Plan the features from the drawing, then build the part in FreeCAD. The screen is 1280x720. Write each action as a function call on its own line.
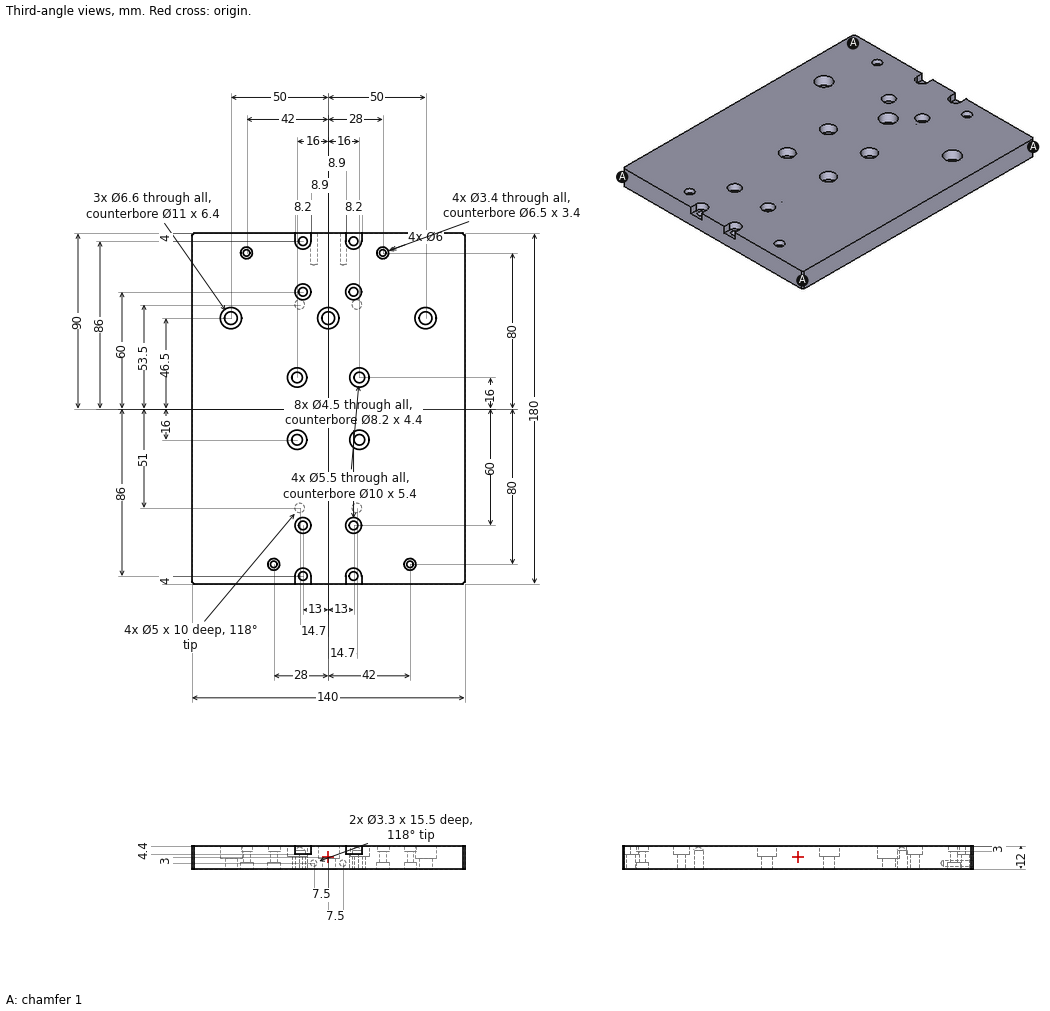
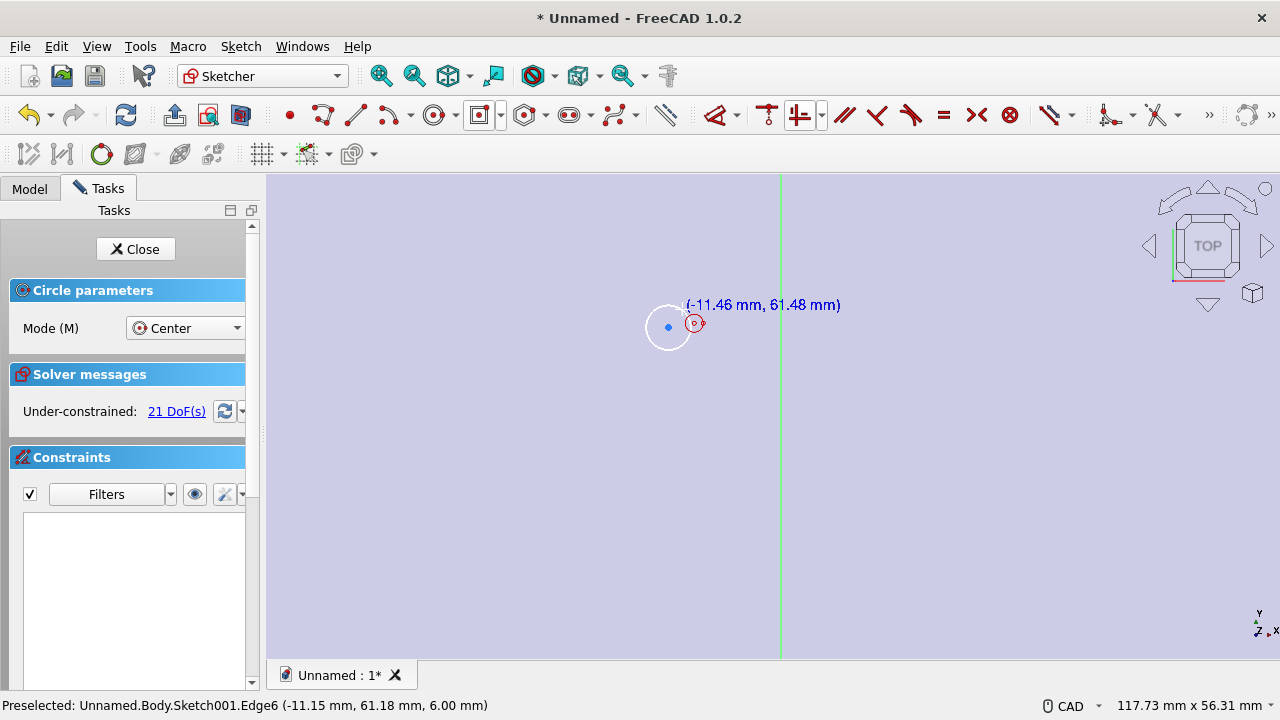
scroll(685, 309, down, 8)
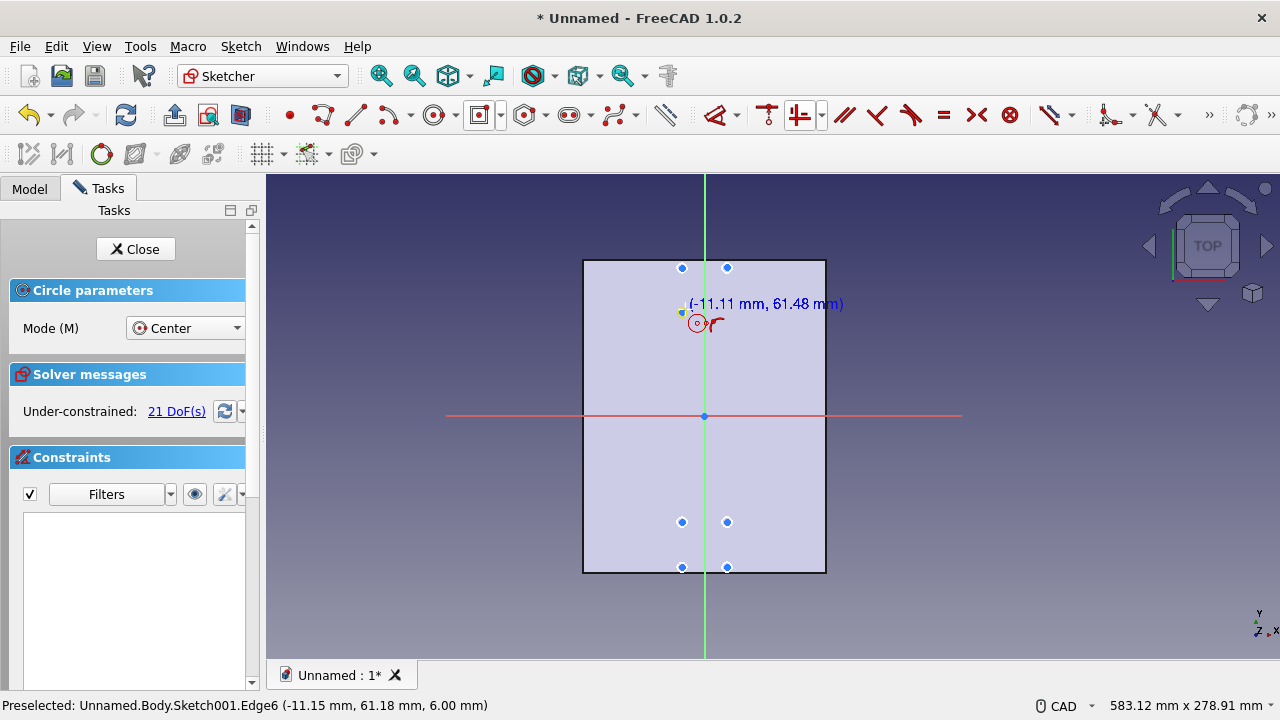
click(727, 312)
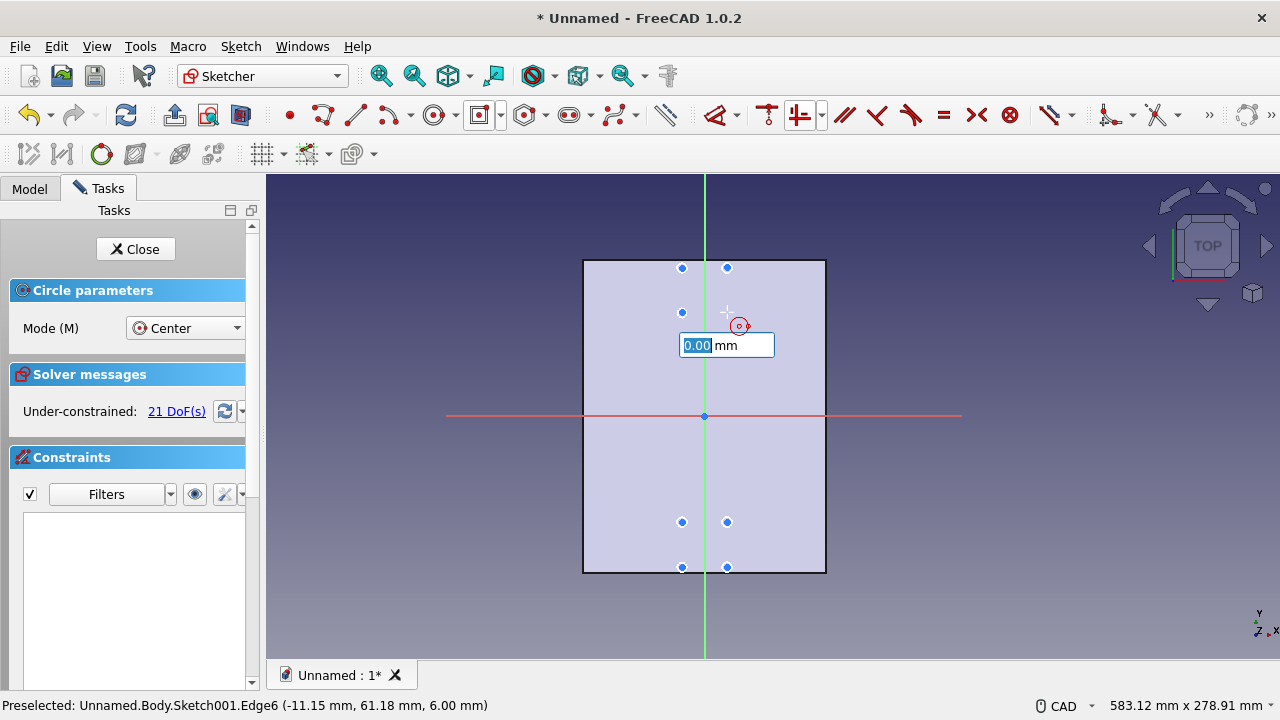
scroll(730, 309, up, 8)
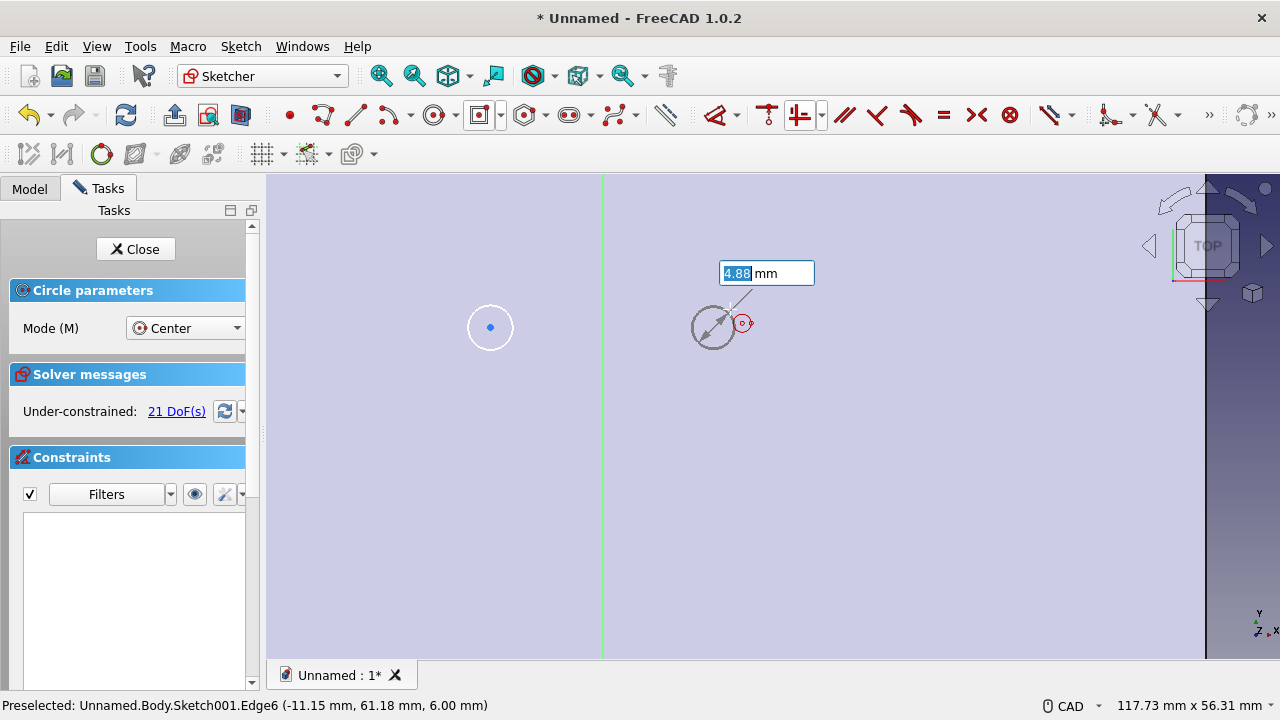
click(728, 309)
key(Escape)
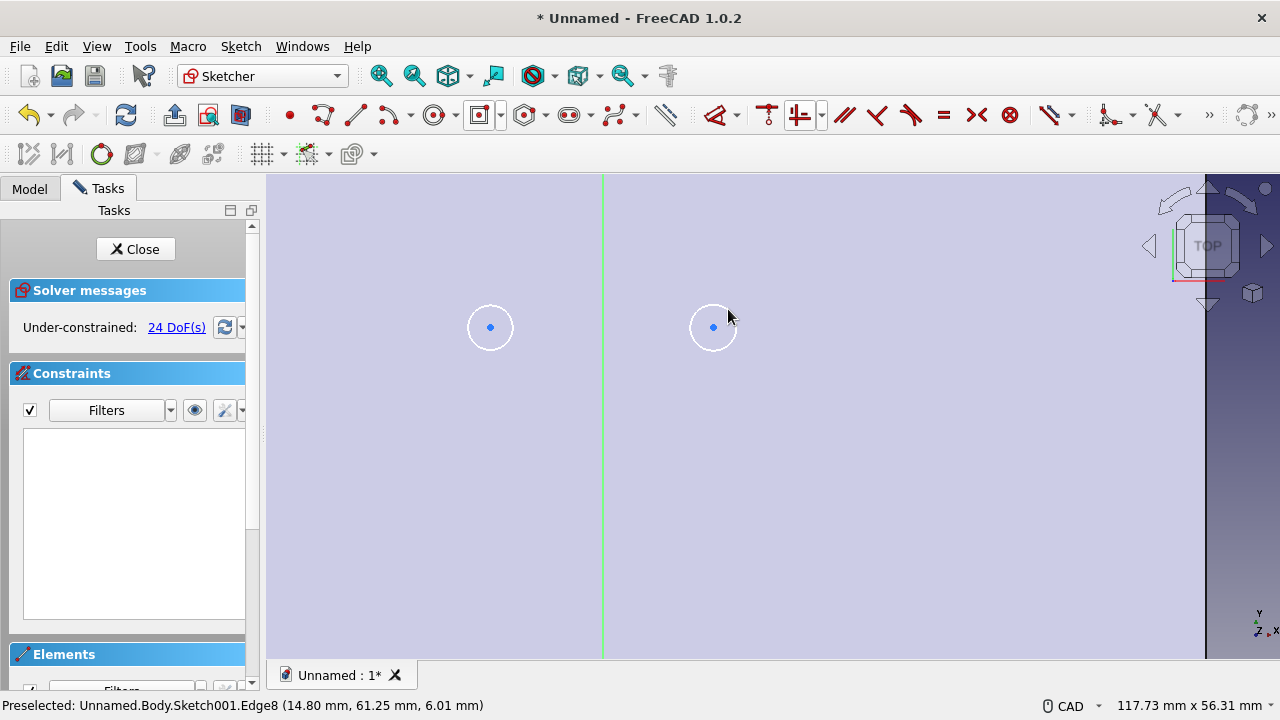
scroll(730, 309, down, 8)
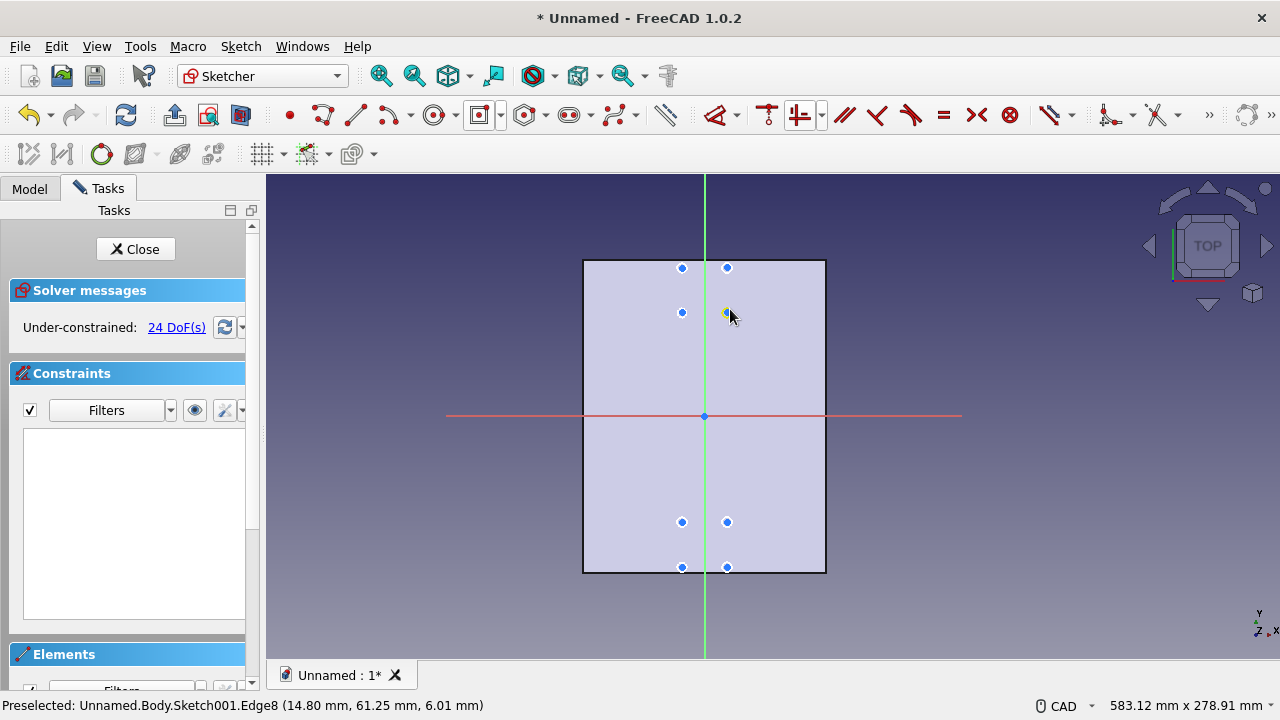
scroll(731, 519, up, 6)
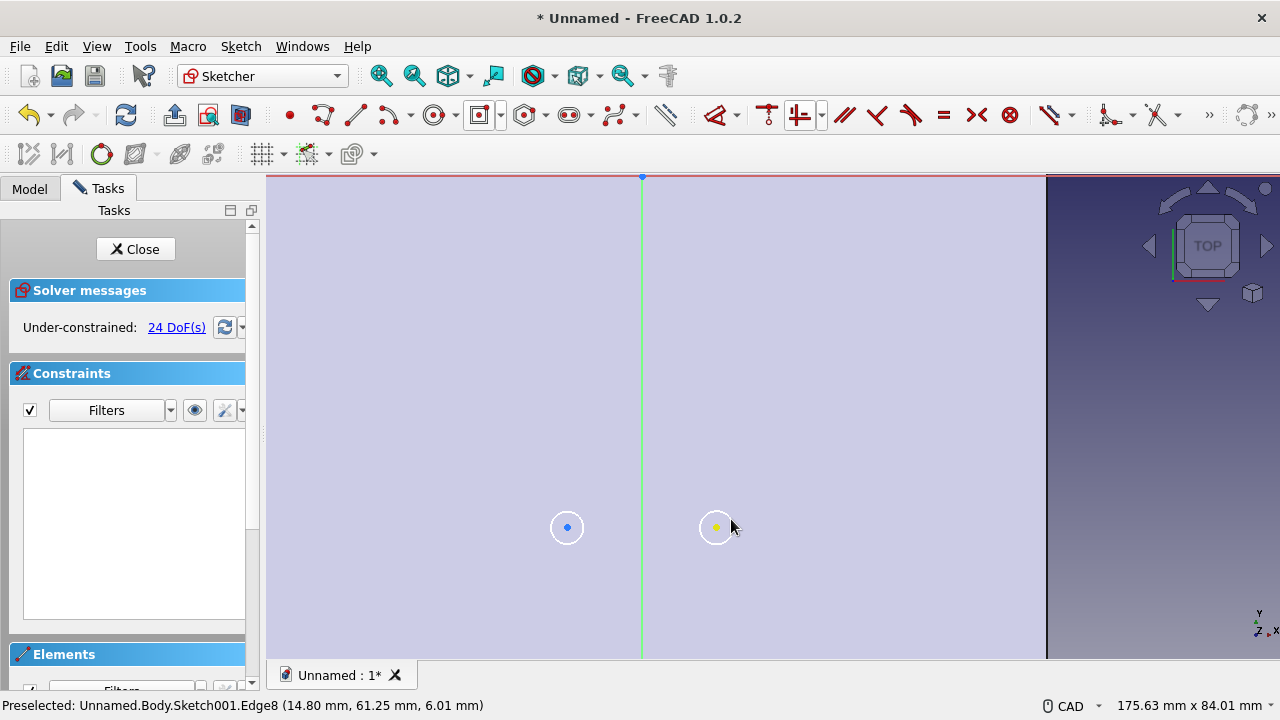
click(728, 516)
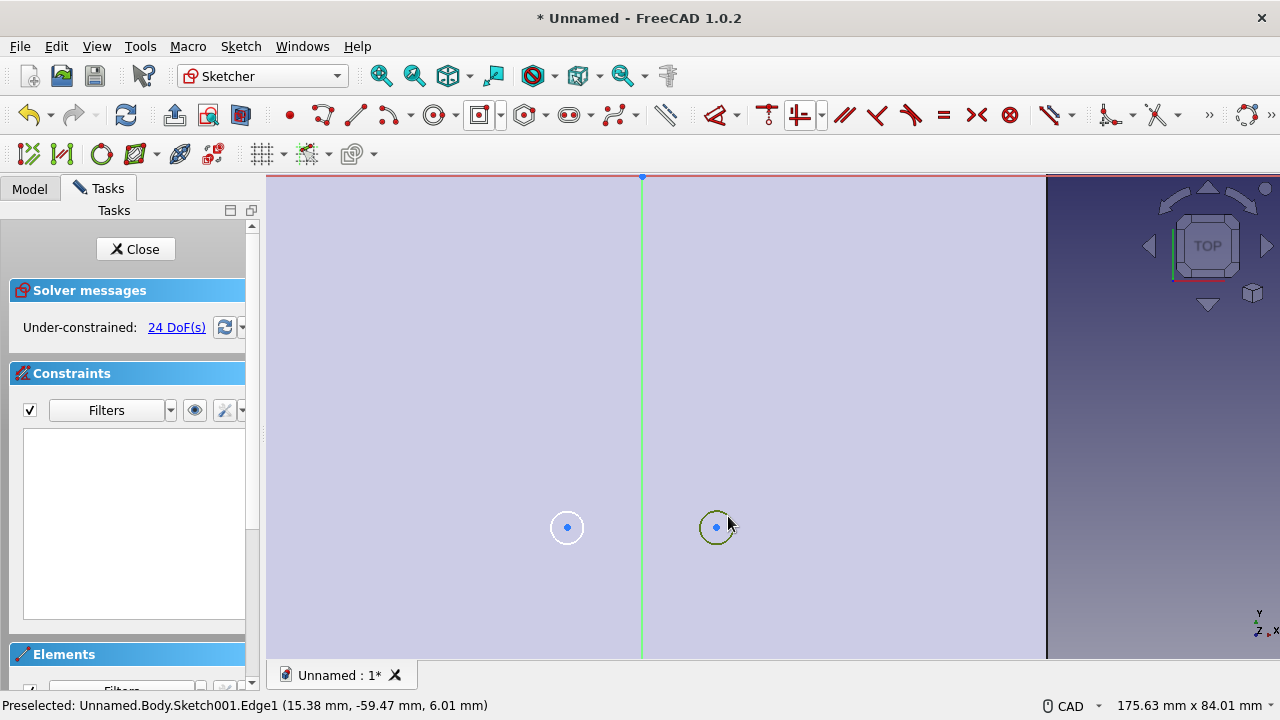
click(579, 516)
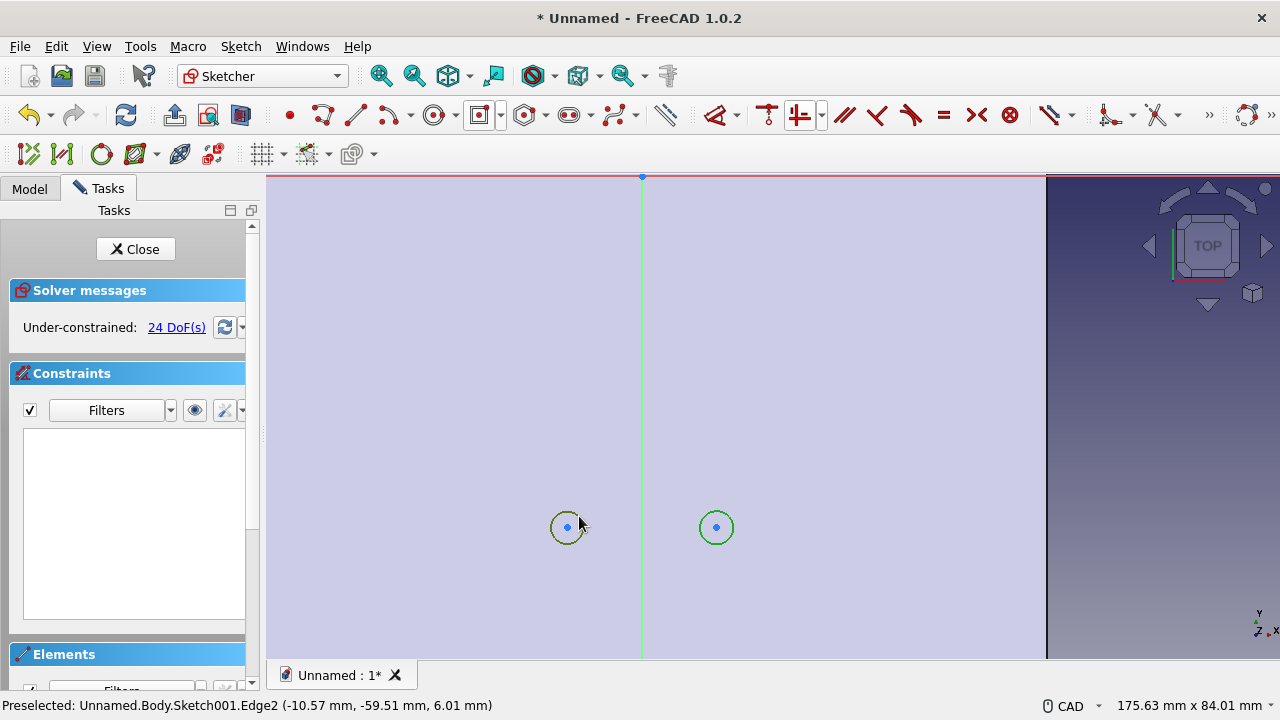
scroll(731, 520, down, 6)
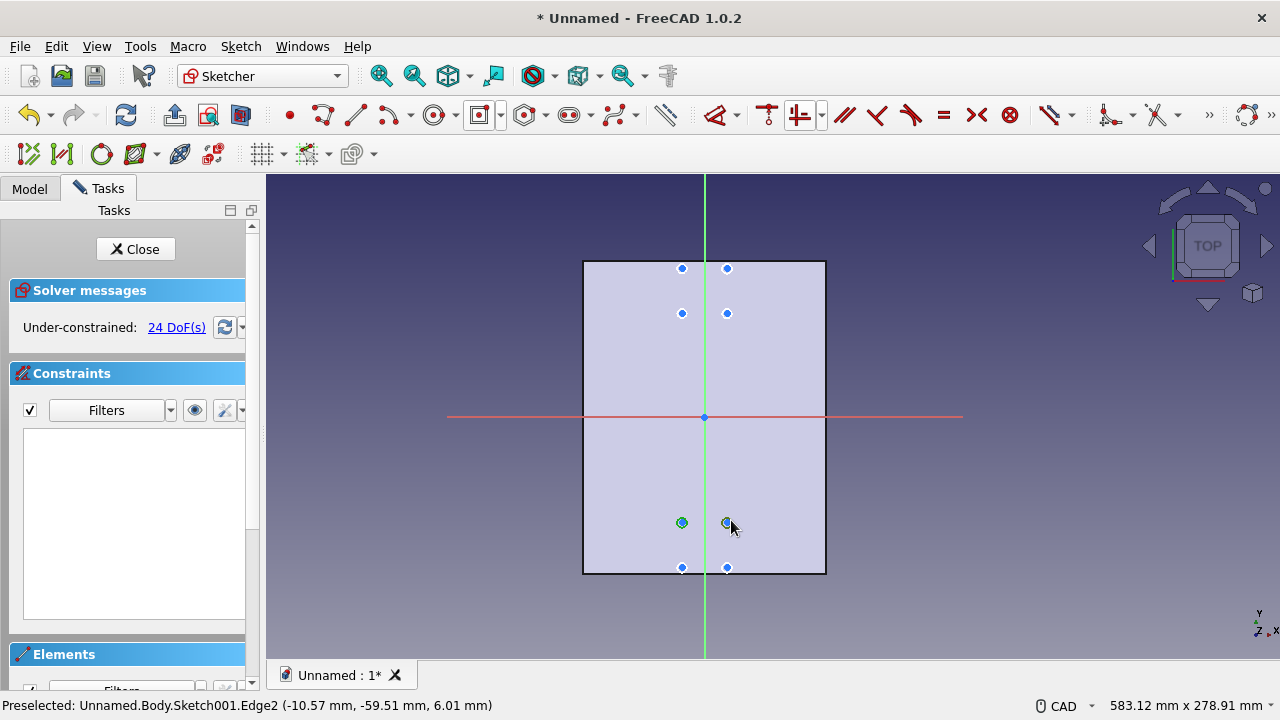
scroll(685, 565, up, 6)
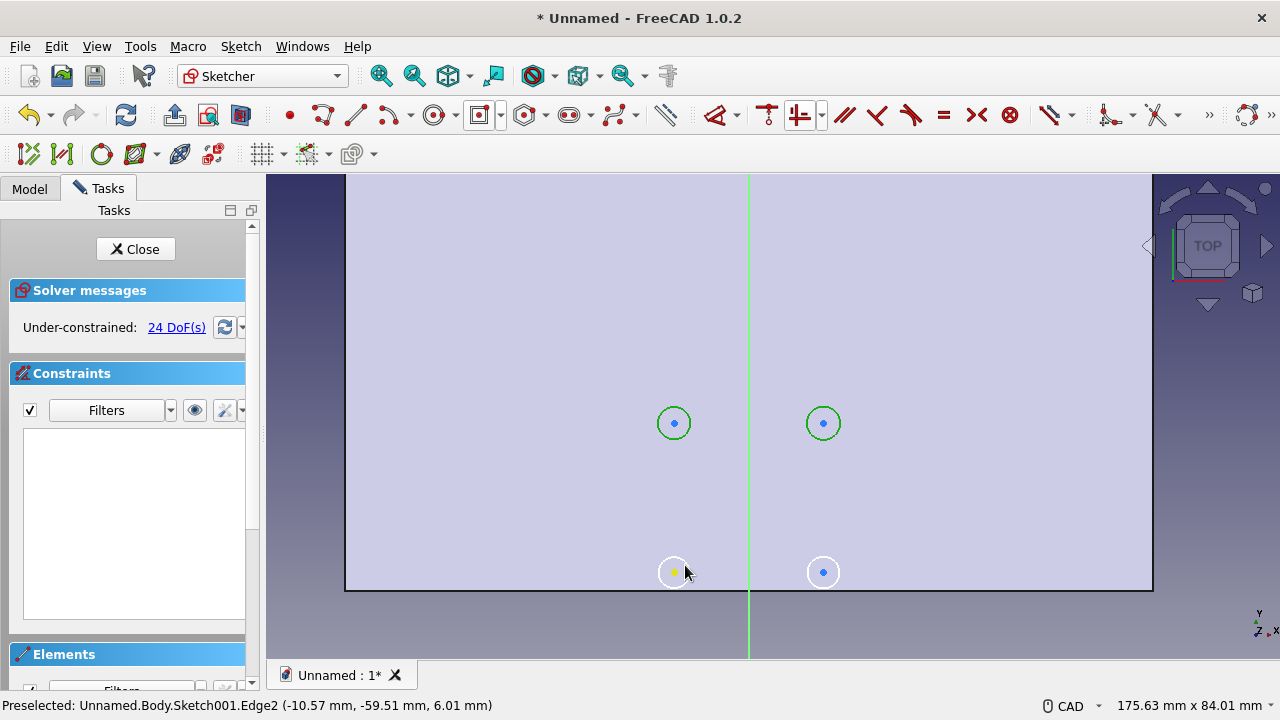
click(685, 562)